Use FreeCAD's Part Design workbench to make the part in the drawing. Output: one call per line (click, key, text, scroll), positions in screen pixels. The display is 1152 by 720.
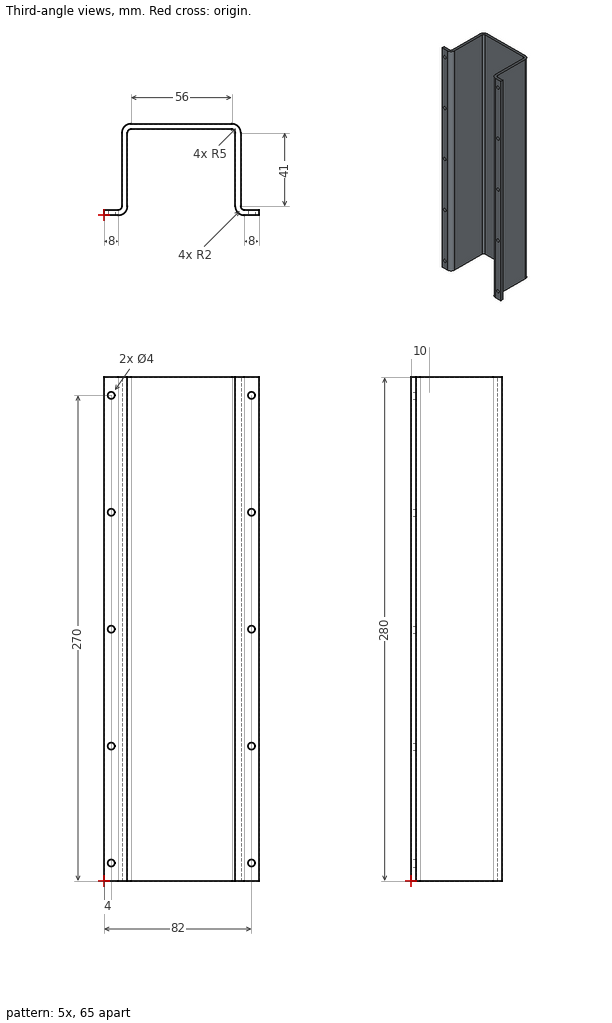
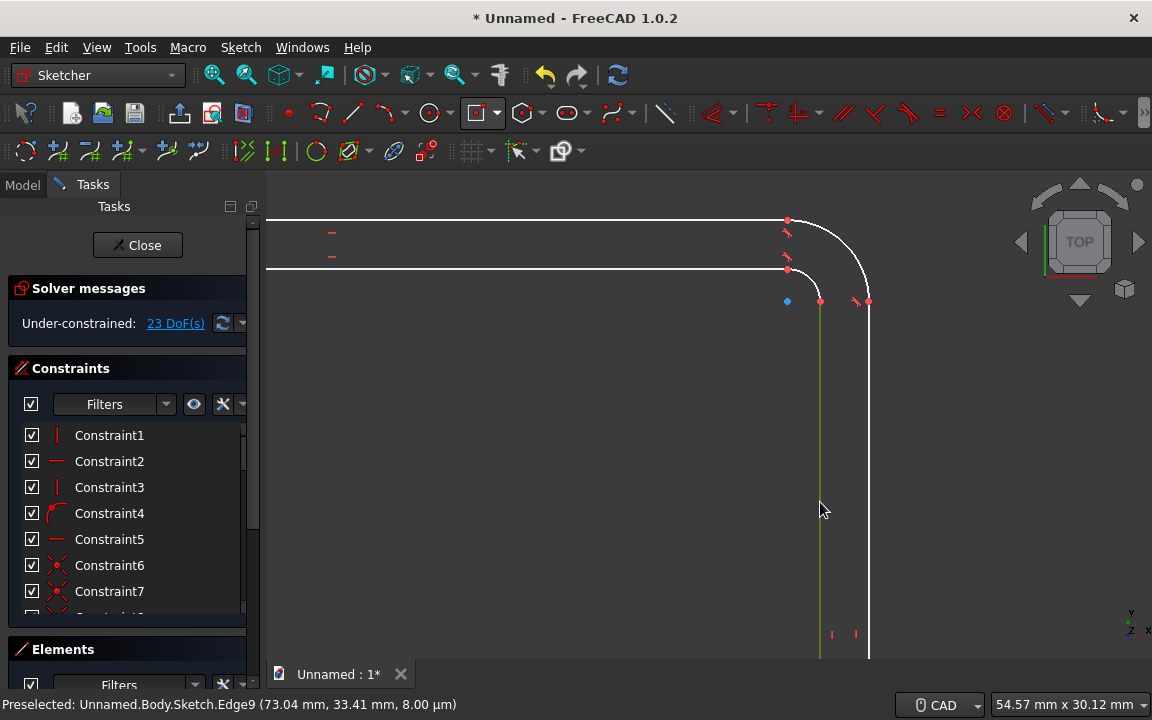
click(817, 287)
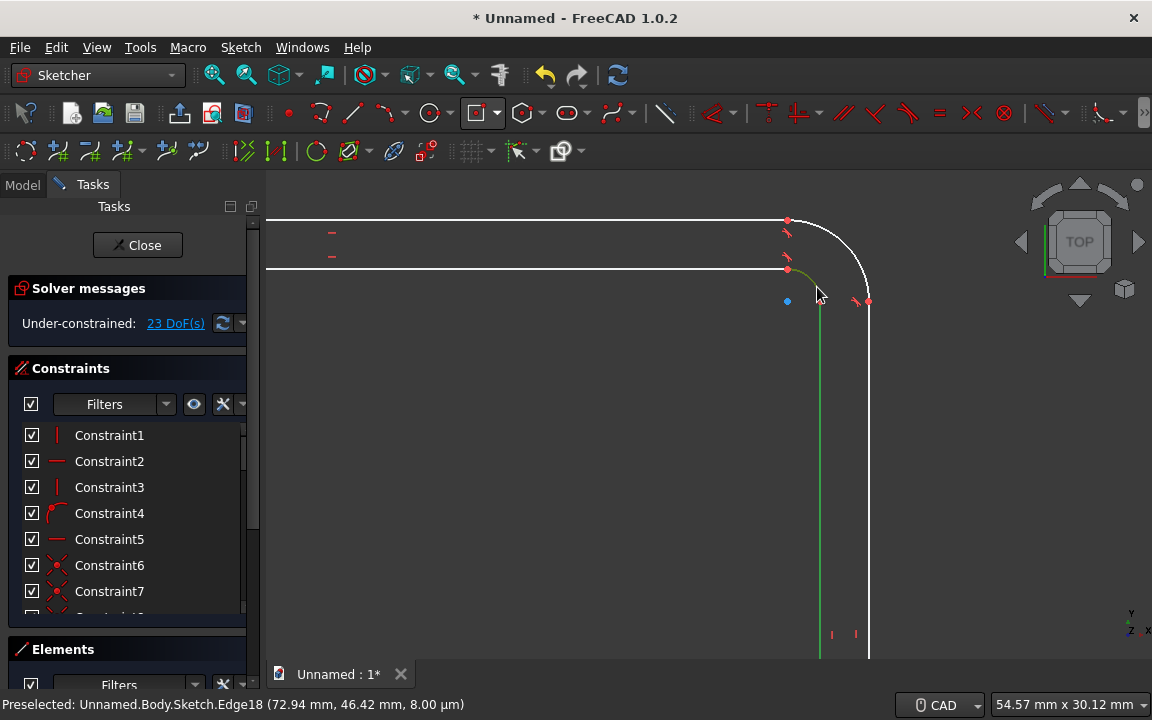
key(t)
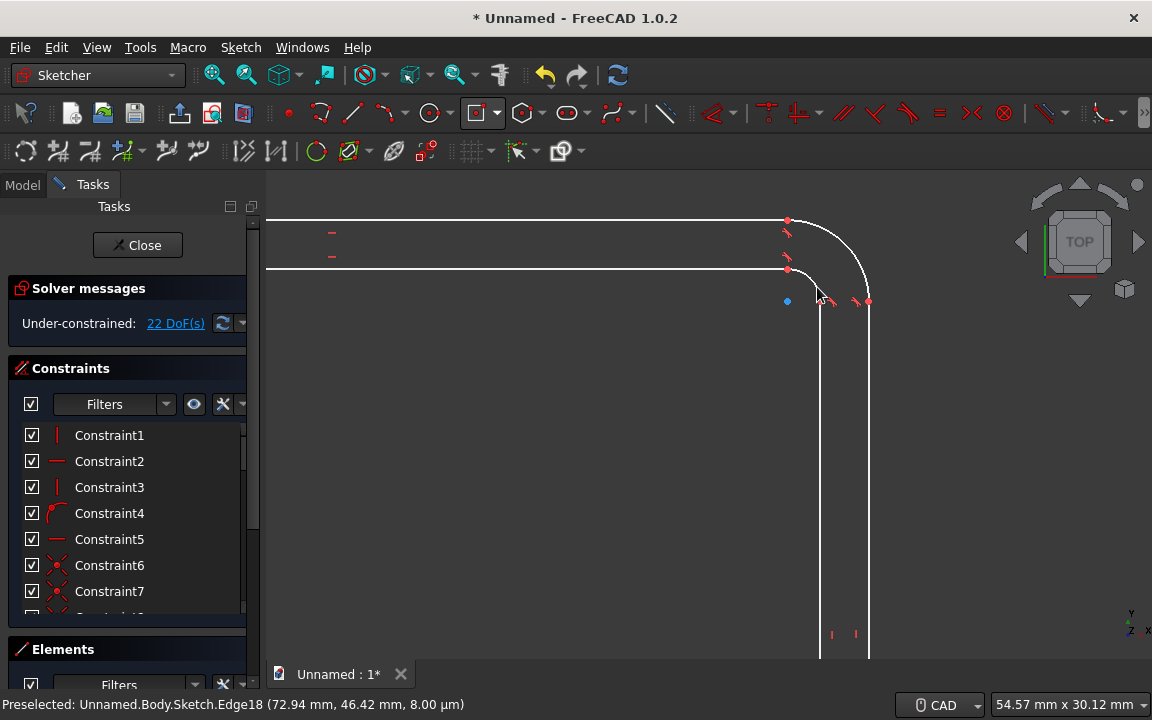
click(820, 502)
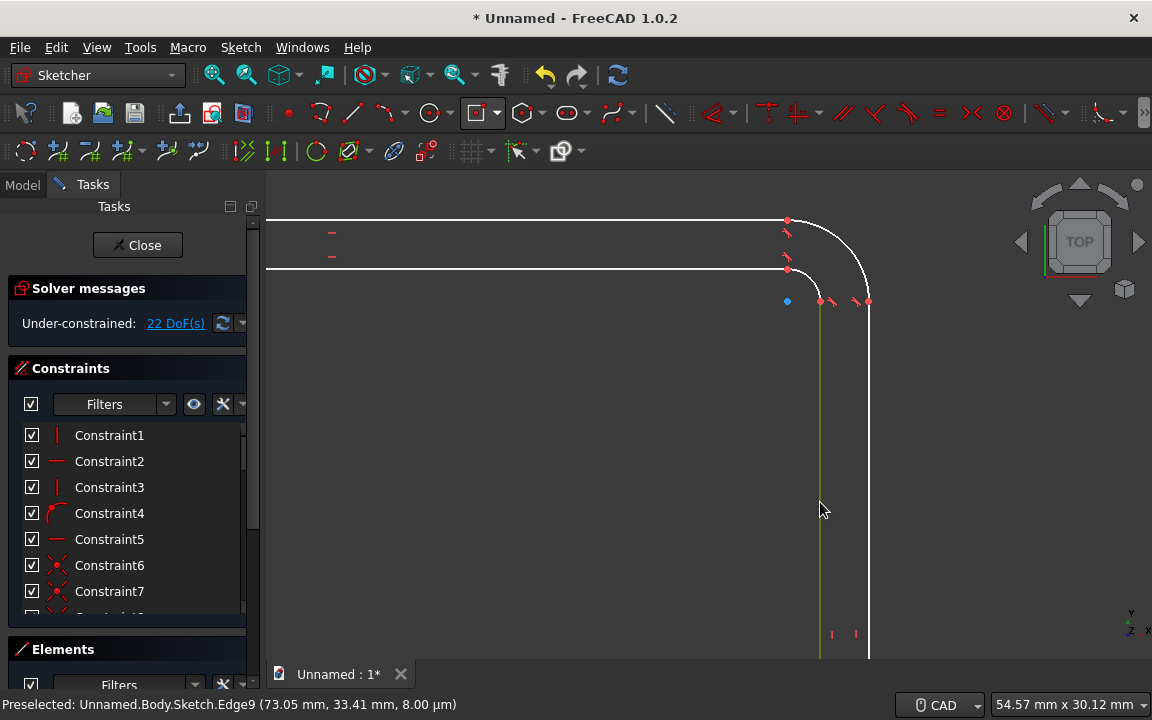
scroll(820, 288, down, 5)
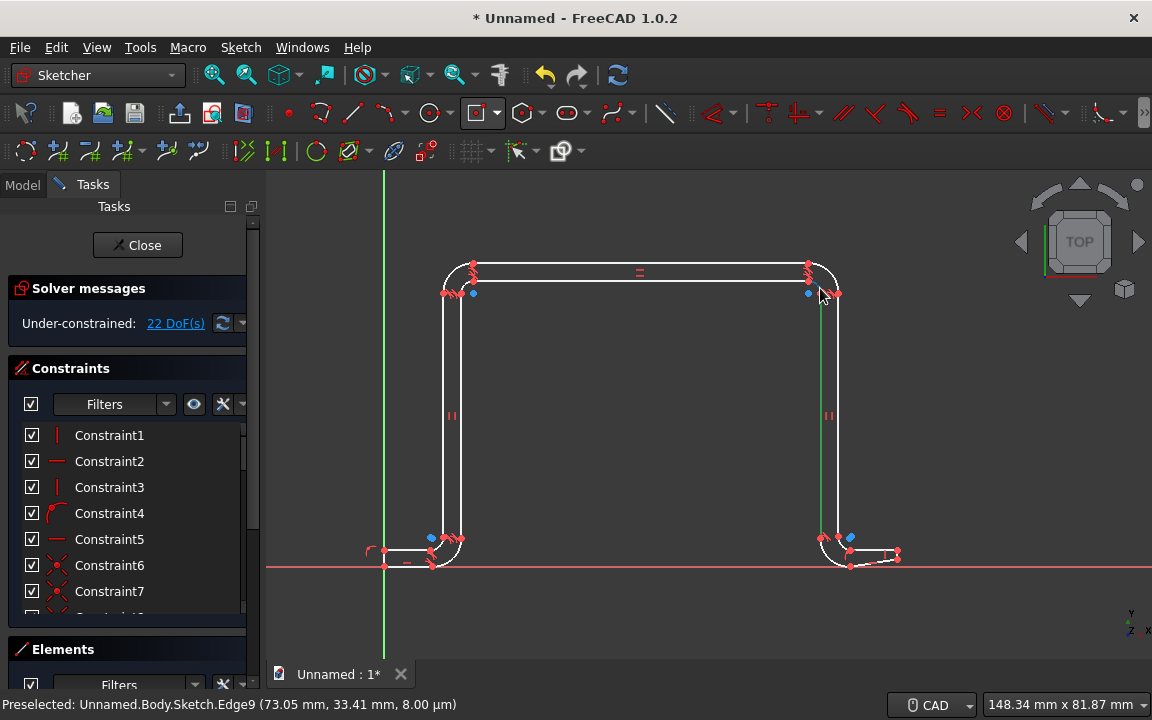
click(824, 552)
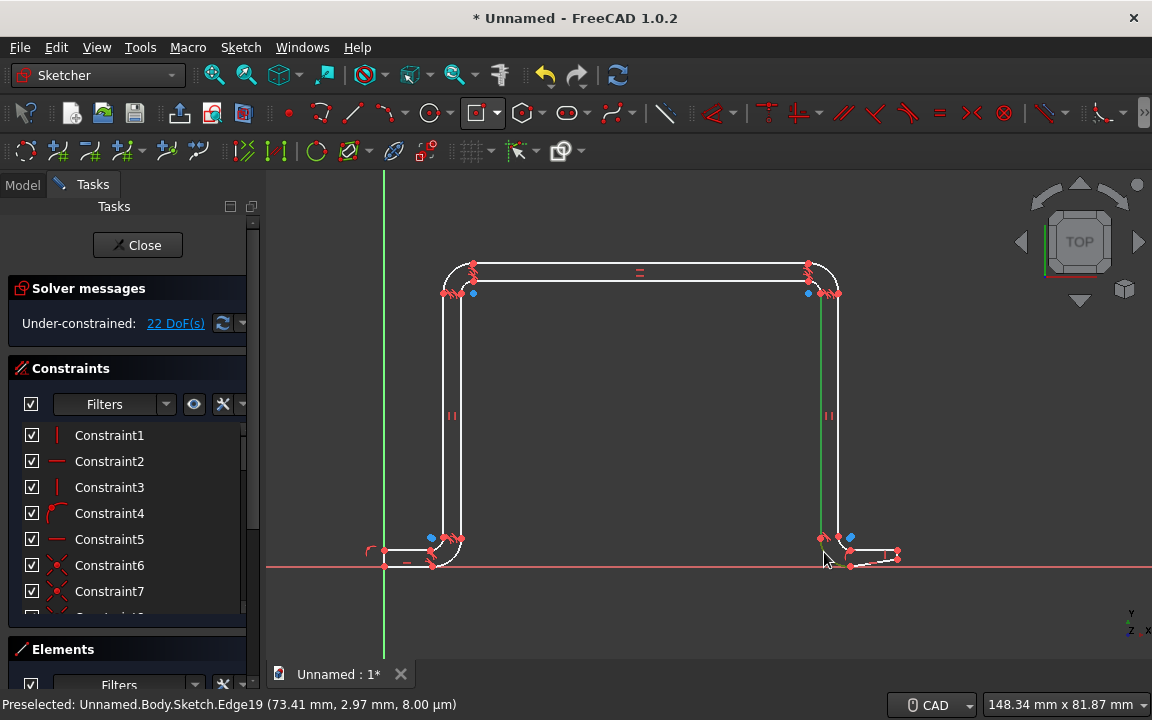
key(t)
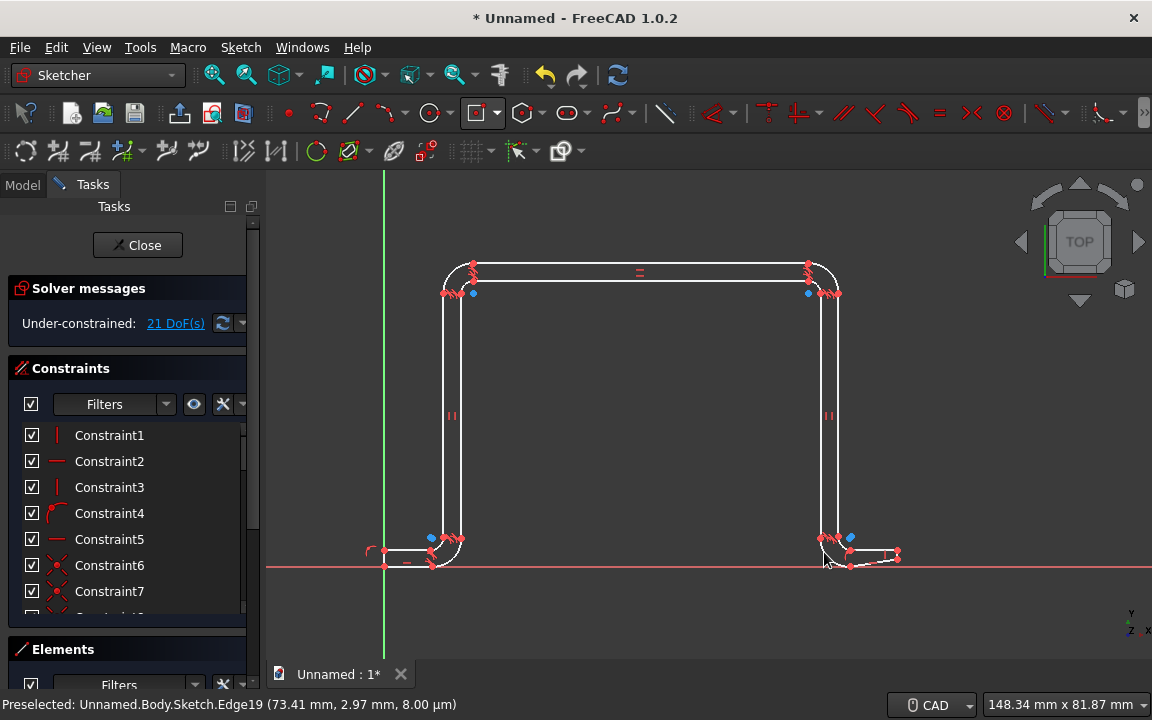
click(865, 565)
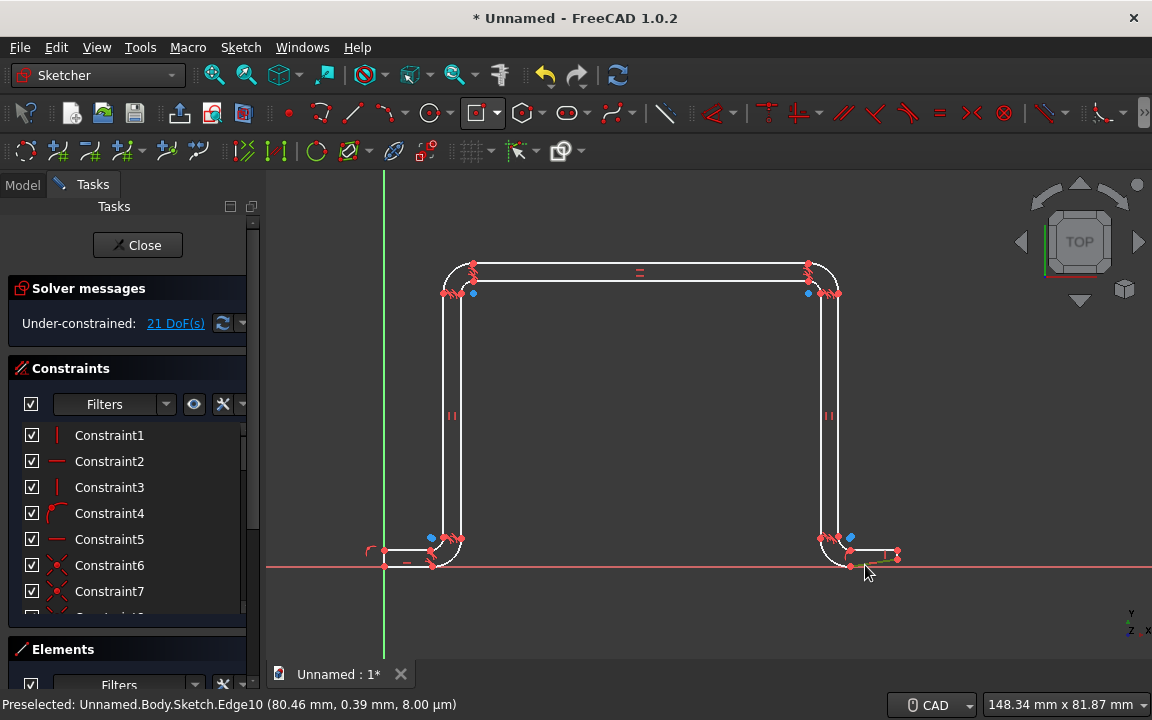
click(824, 551)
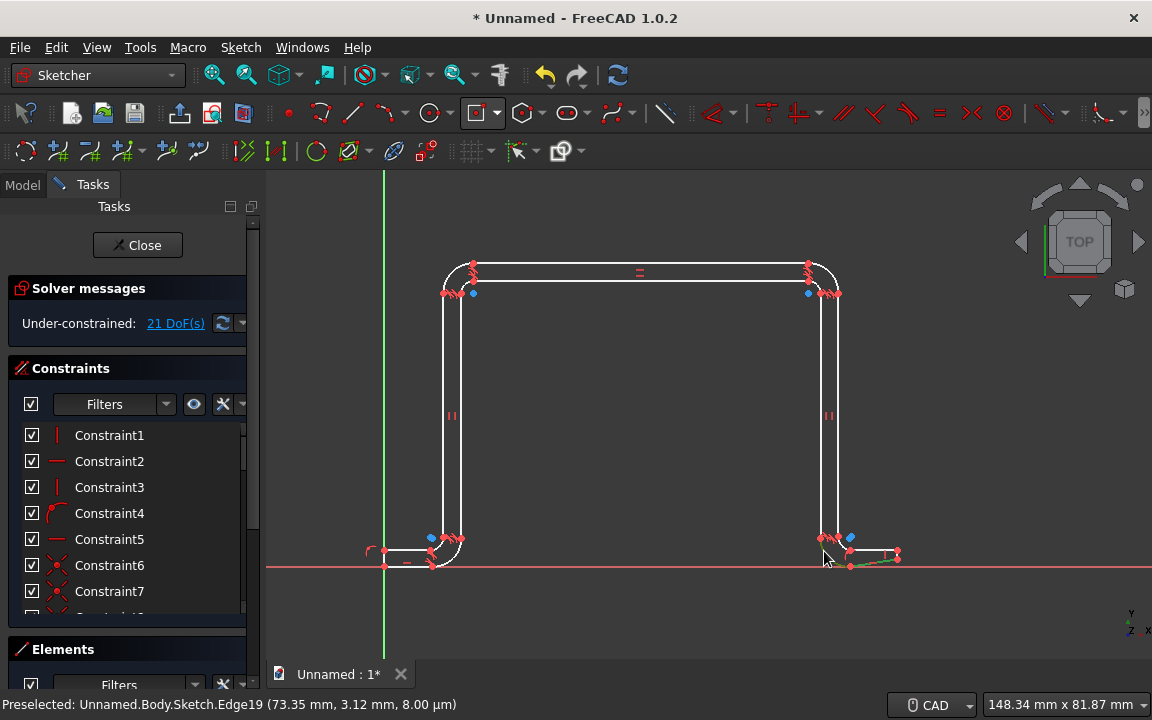
key(t)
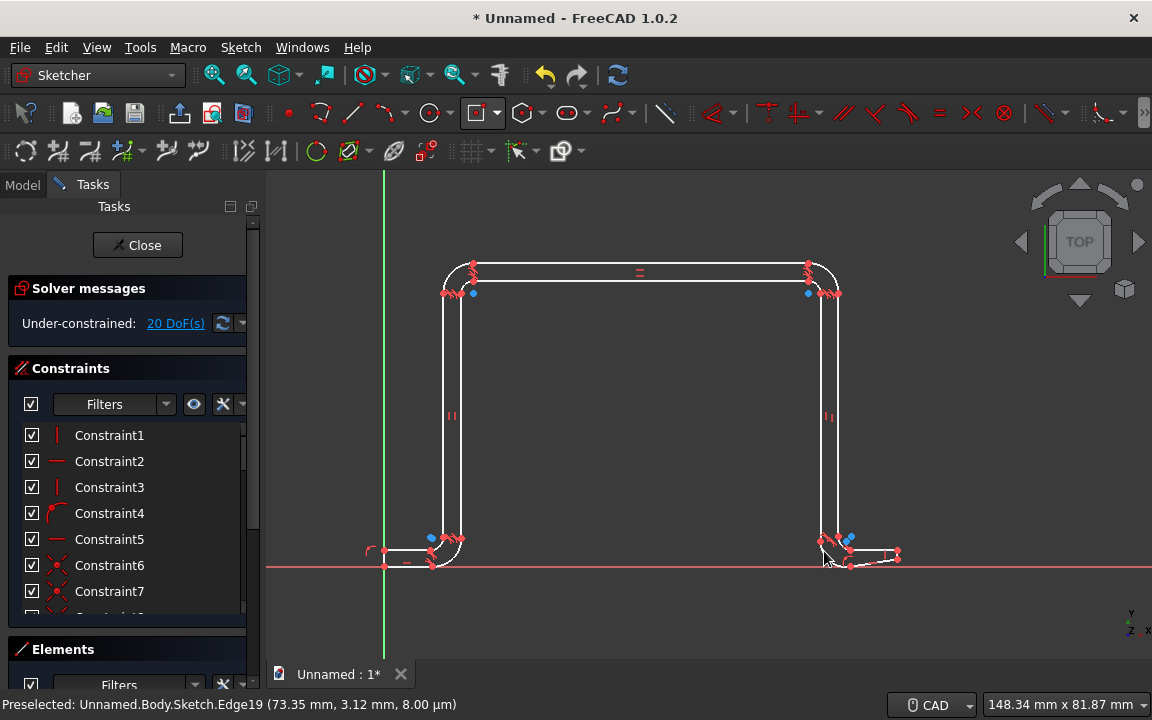
scroll(883, 550, up, 2)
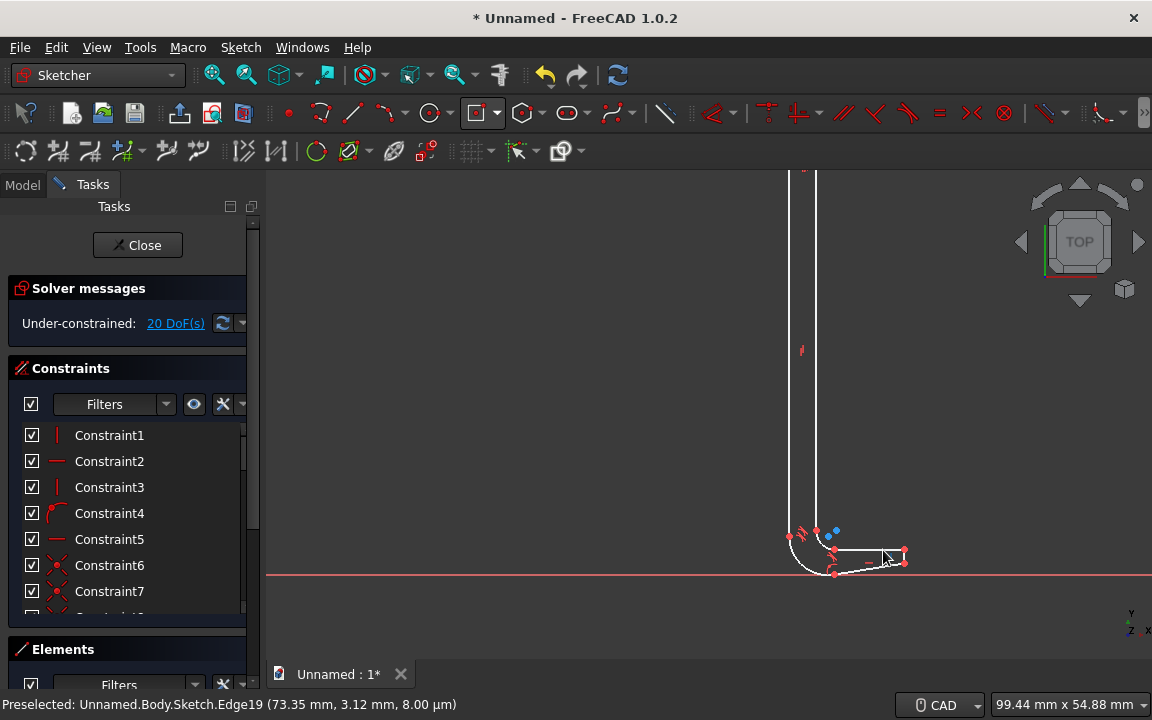
click(883, 550)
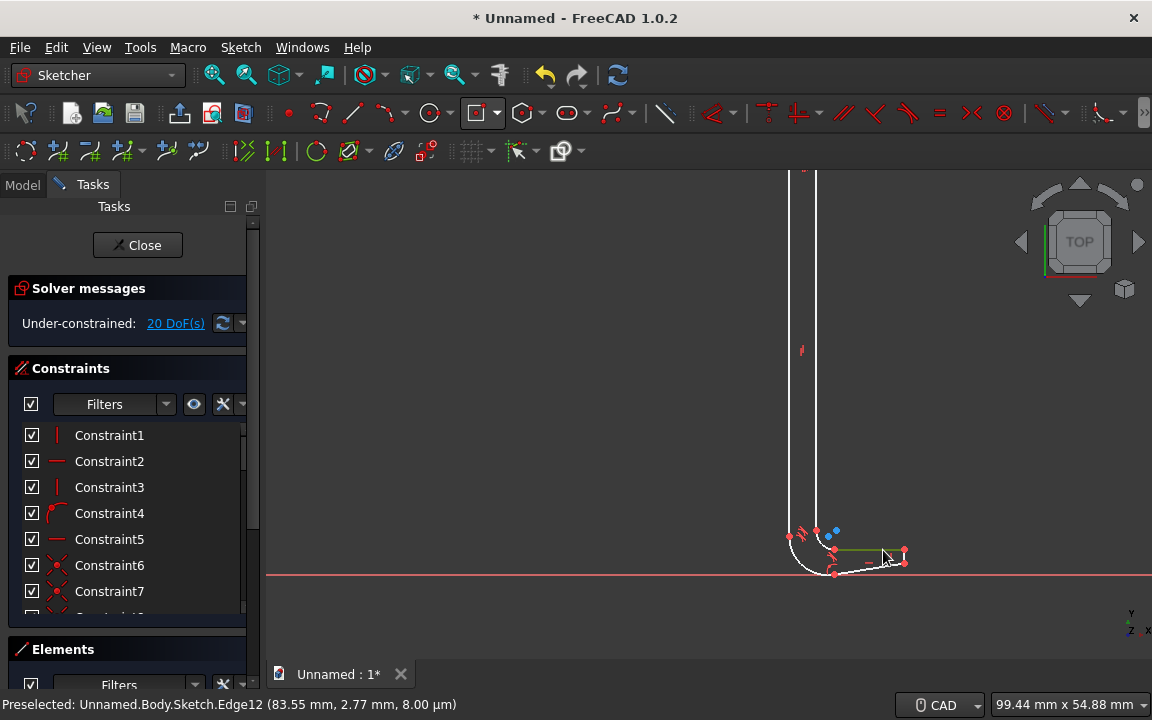
click(821, 544)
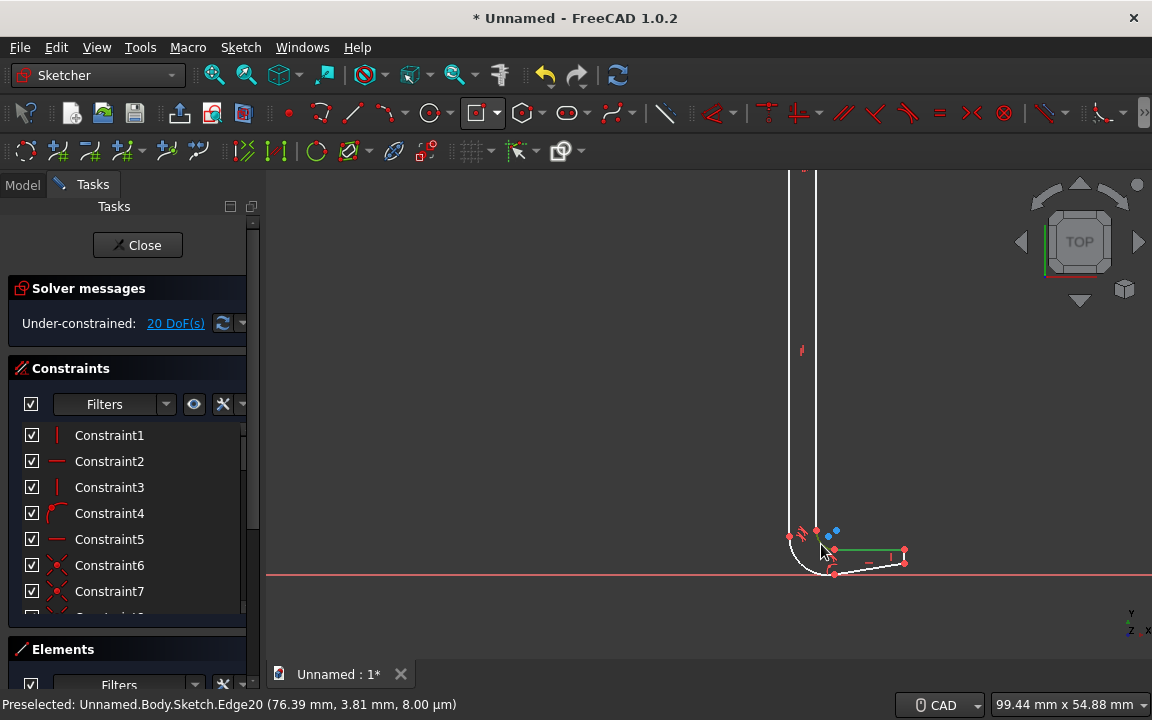
click(908, 114)